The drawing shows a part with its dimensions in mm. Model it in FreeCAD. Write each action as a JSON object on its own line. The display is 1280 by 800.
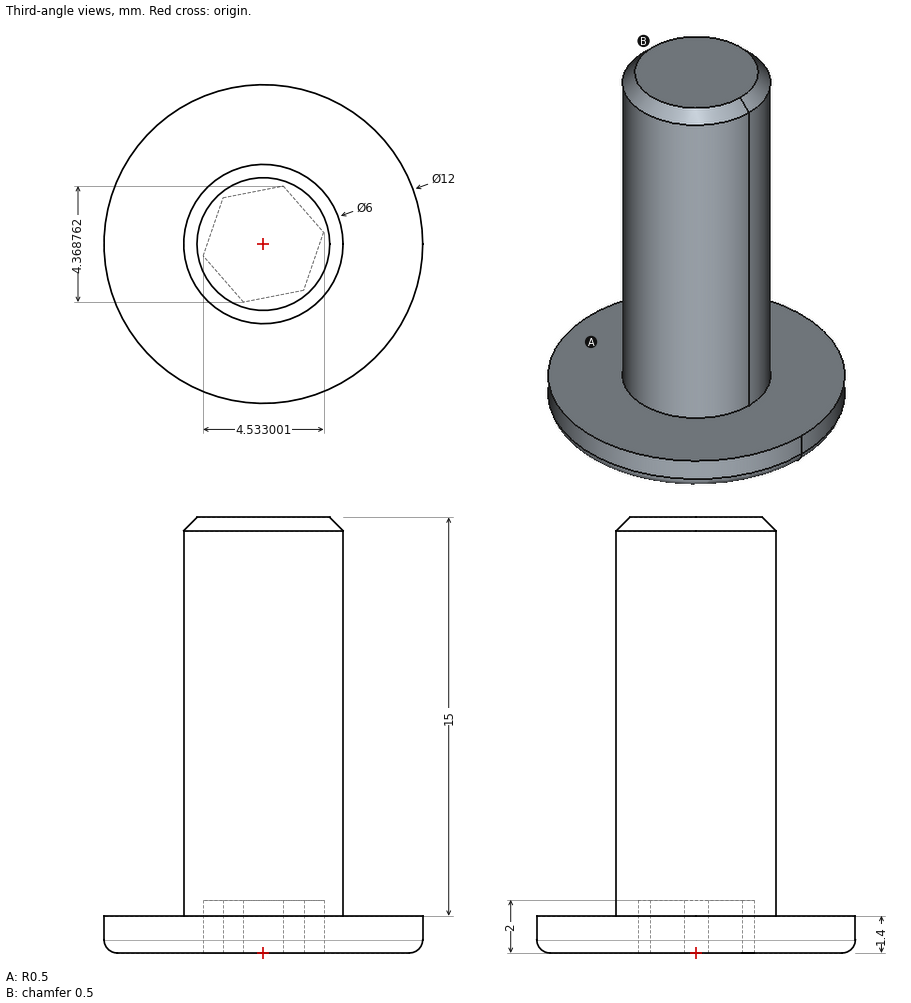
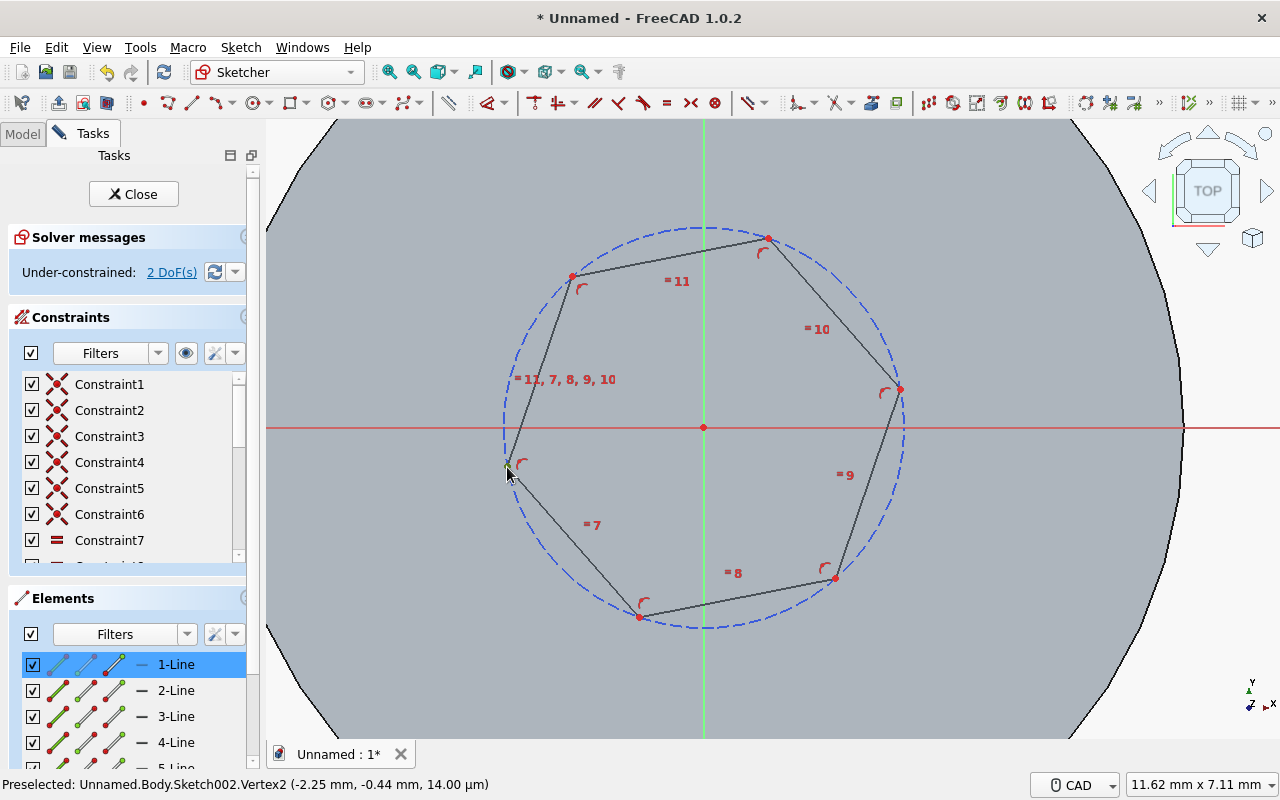
{"action": "left_click", "coordinate": [900, 389]}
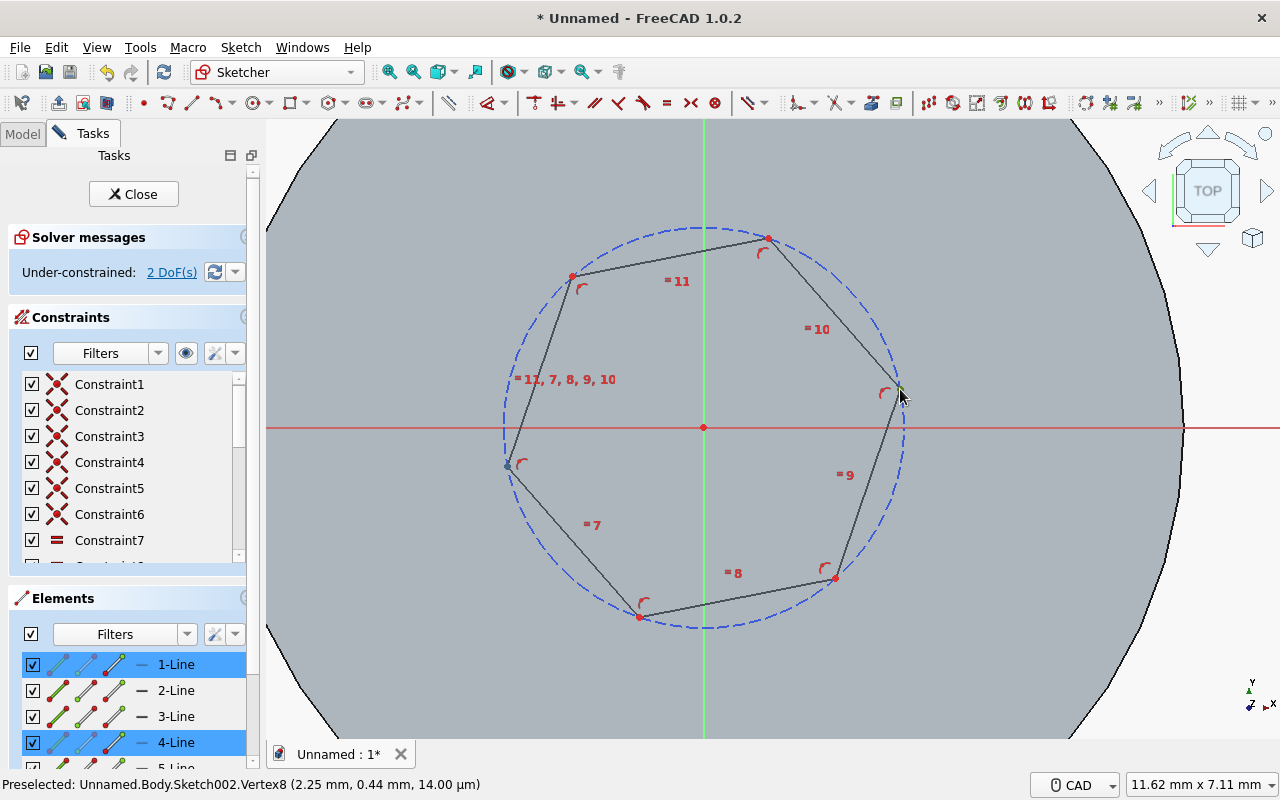
{"action": "key", "text": "l"}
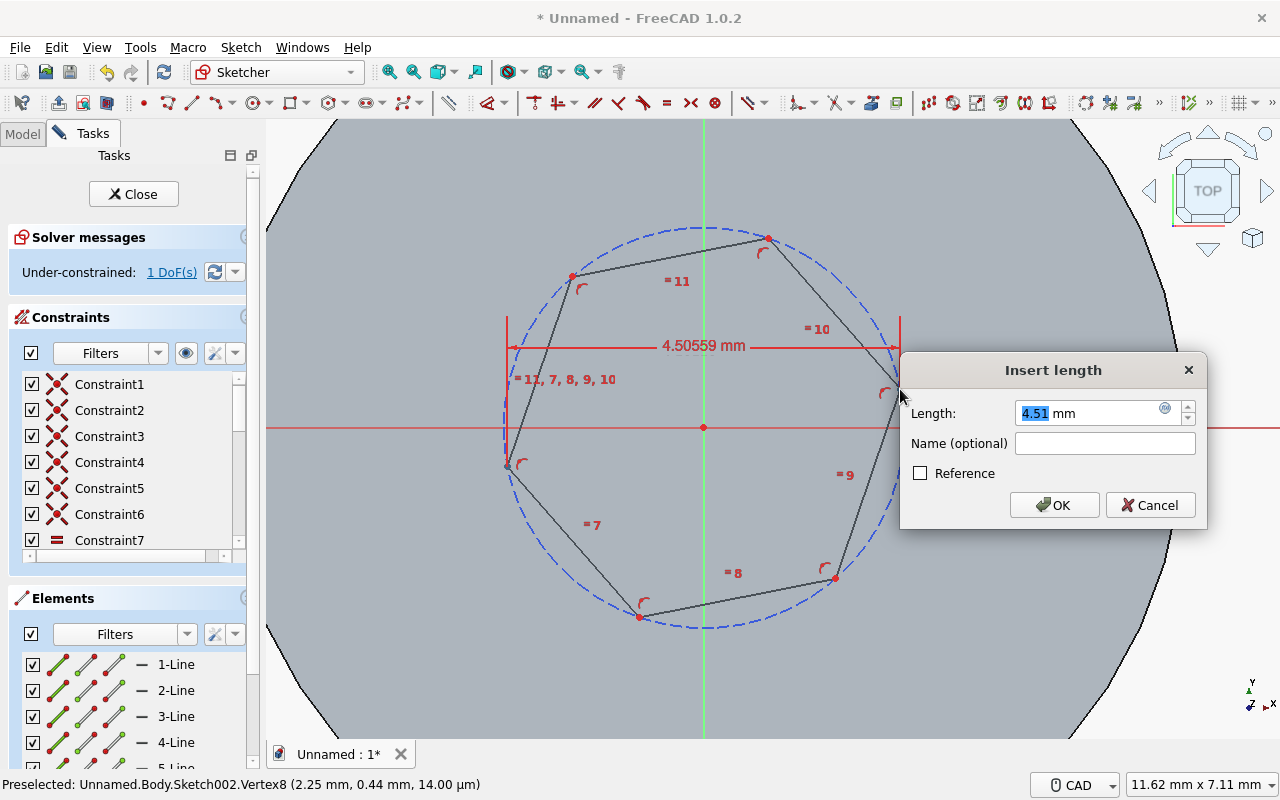
{"action": "type", "text": "4.533001"}
{"action": "key", "text": "Return"}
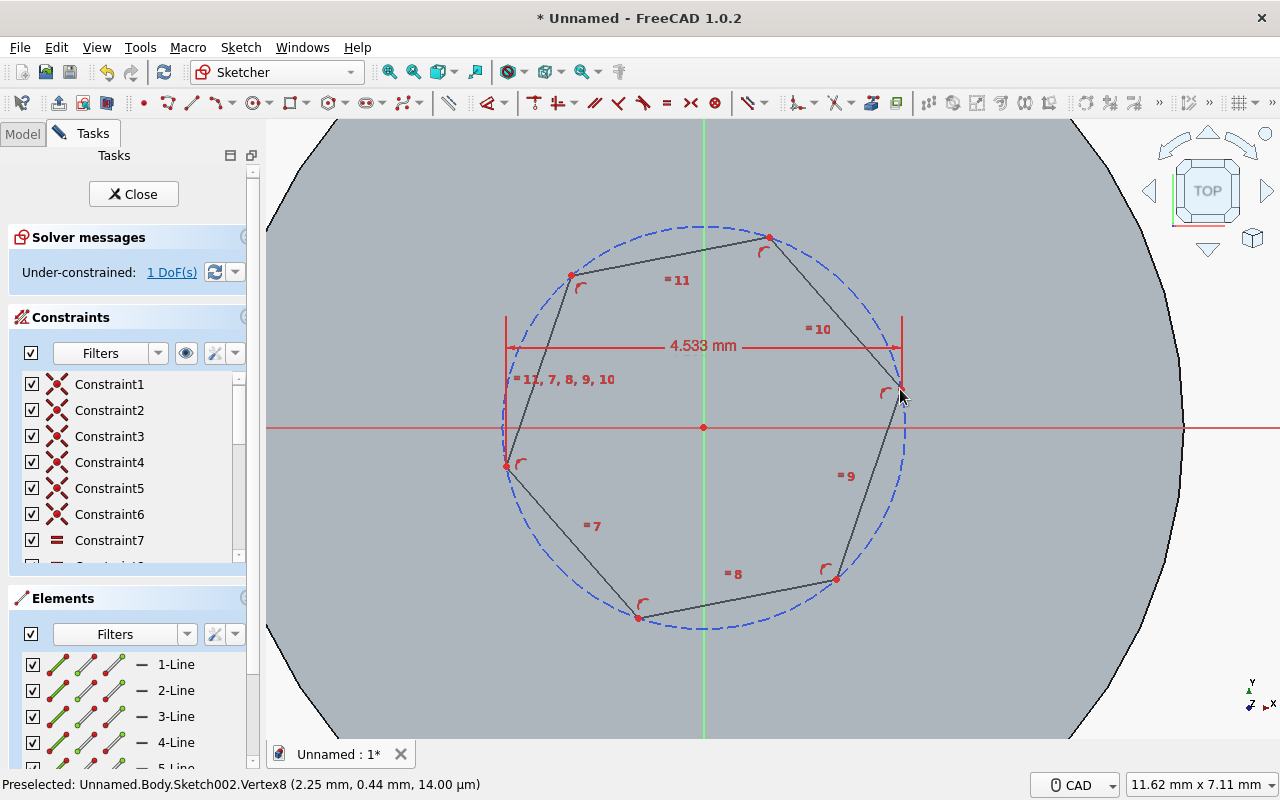
{"action": "left_click", "coordinate": [639, 619]}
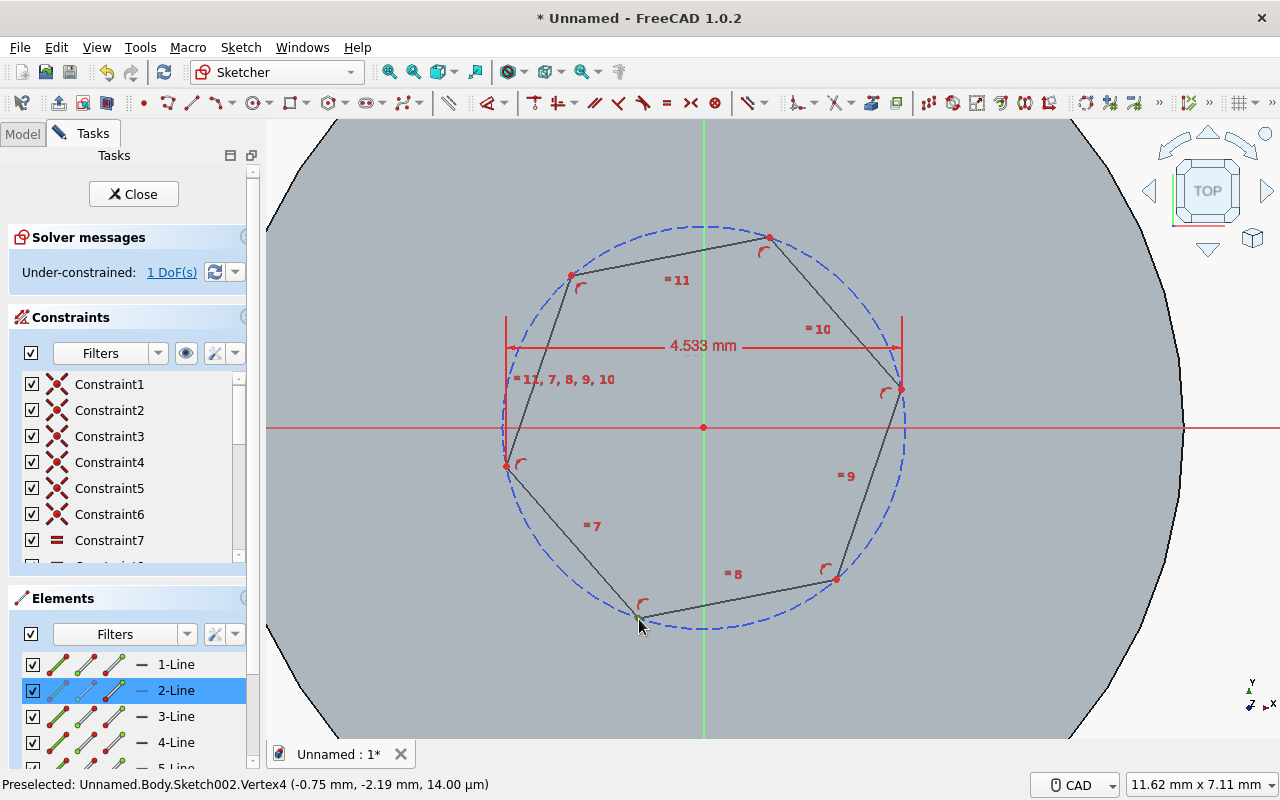
{"action": "left_click", "coordinate": [769, 237]}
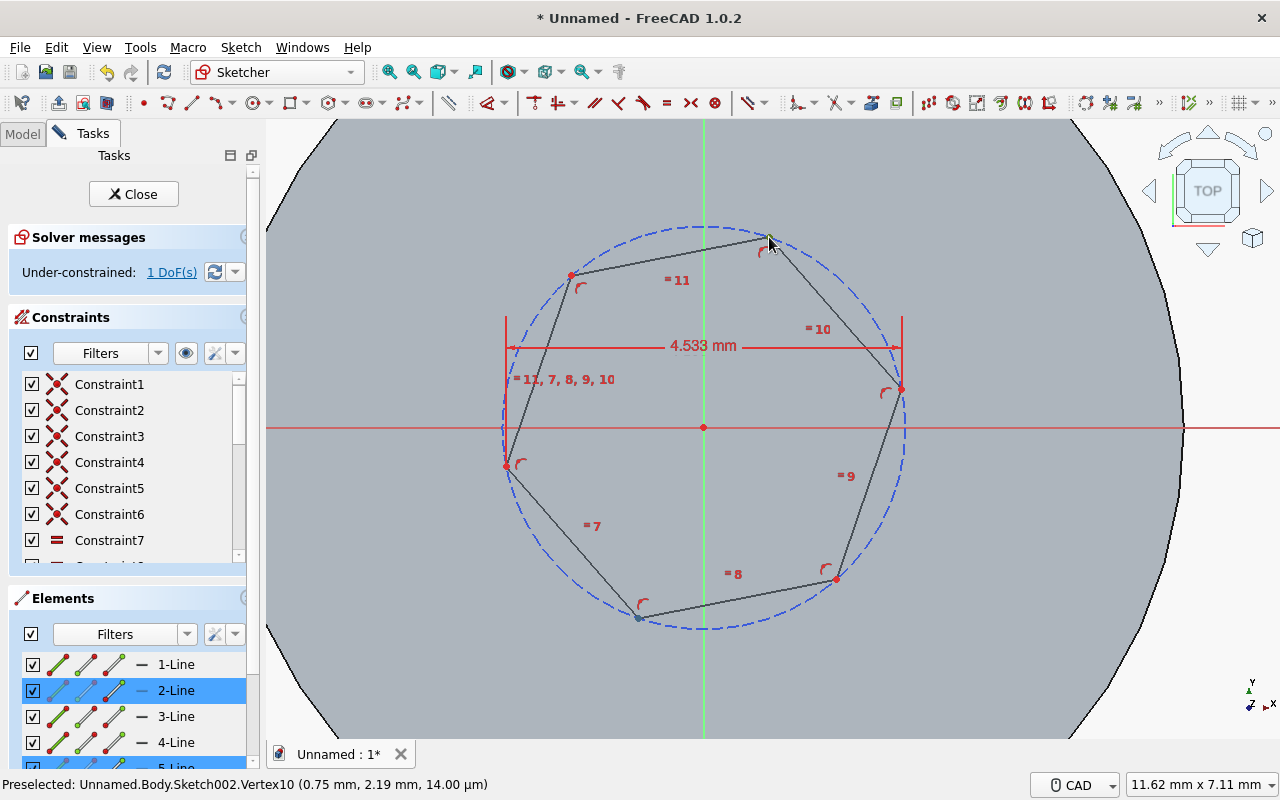
{"action": "left_click", "coordinate": [506, 104]}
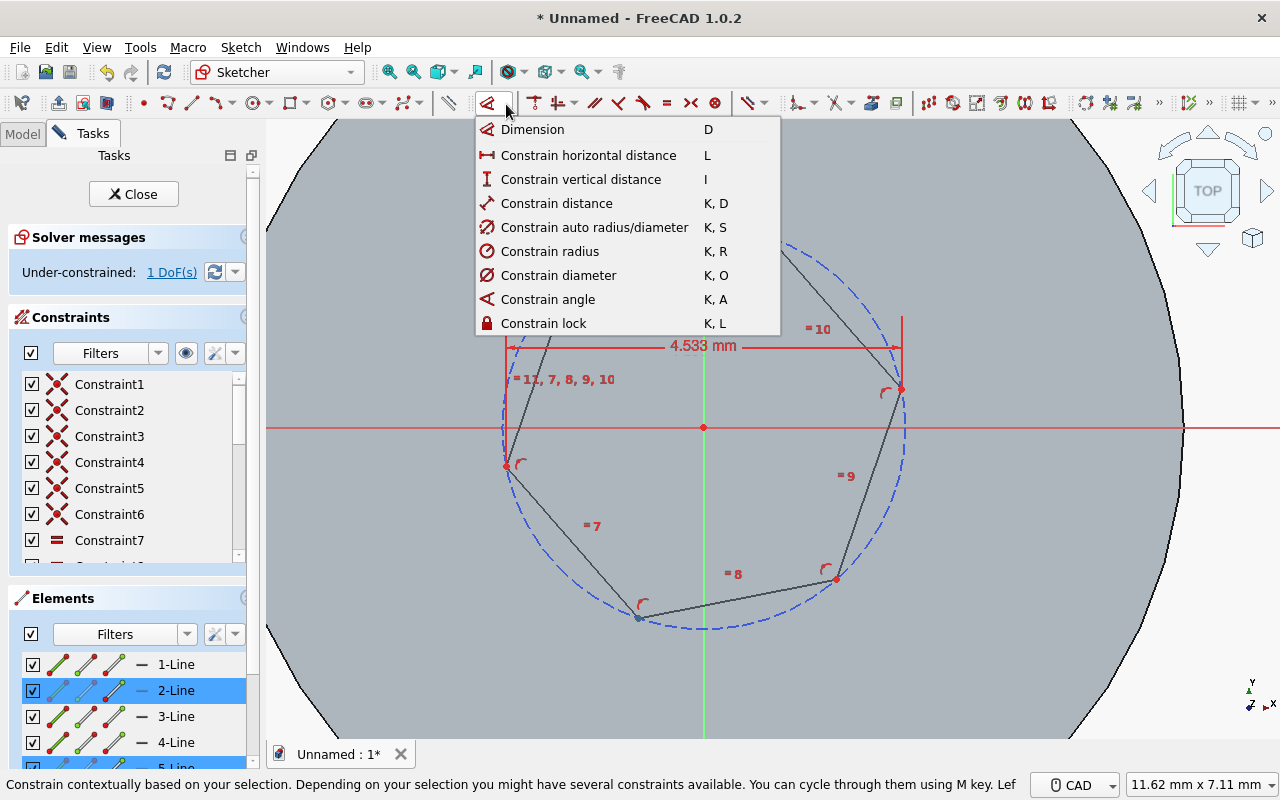
{"action": "left_click", "coordinate": [628, 179]}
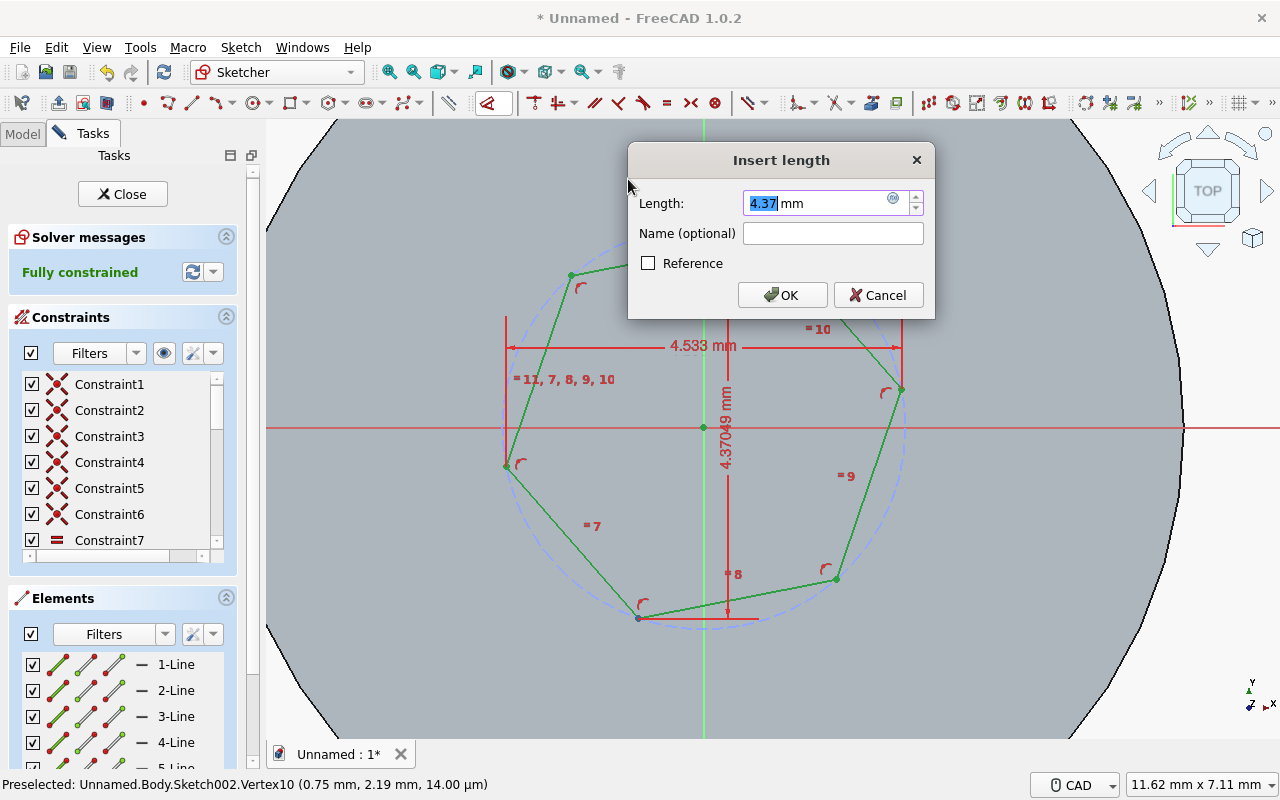
{"action": "type", "text": "4.368762"}
{"action": "key", "text": "Return"}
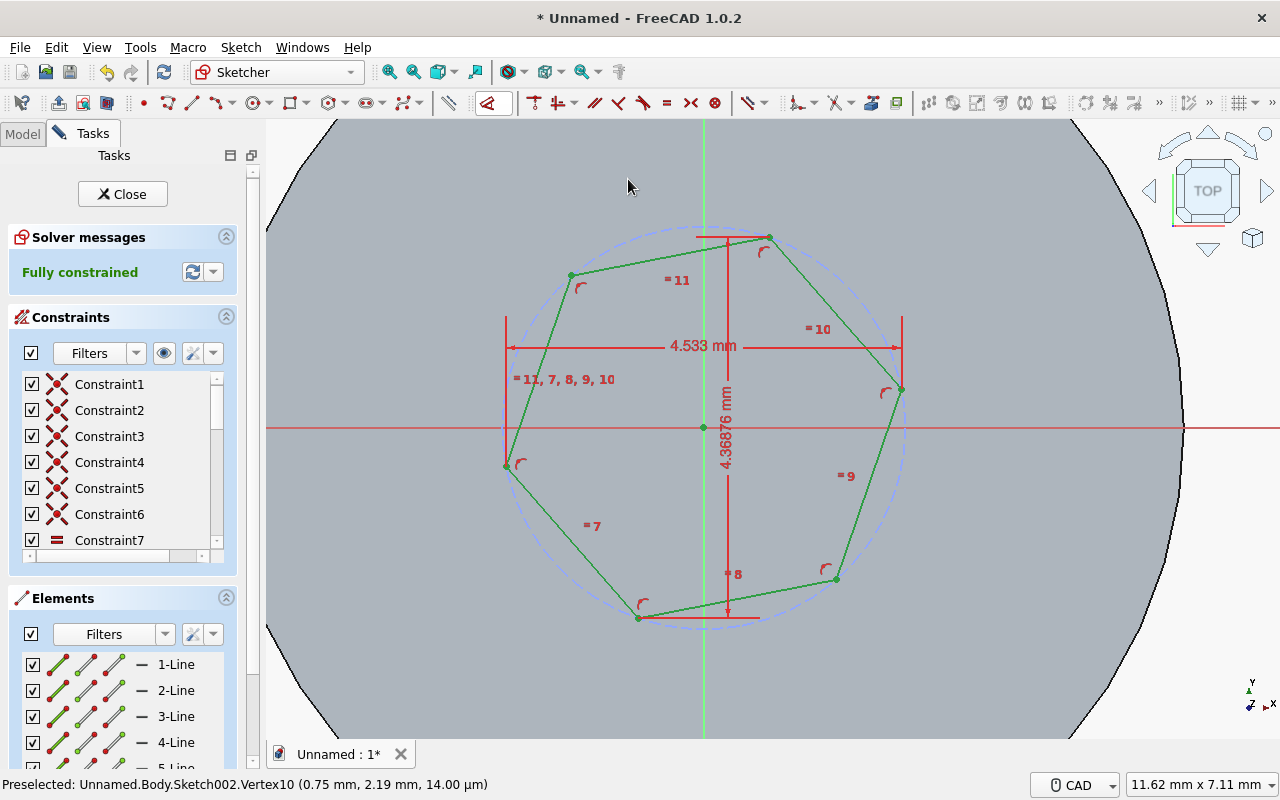
{"action": "left_click", "coordinate": [123, 194]}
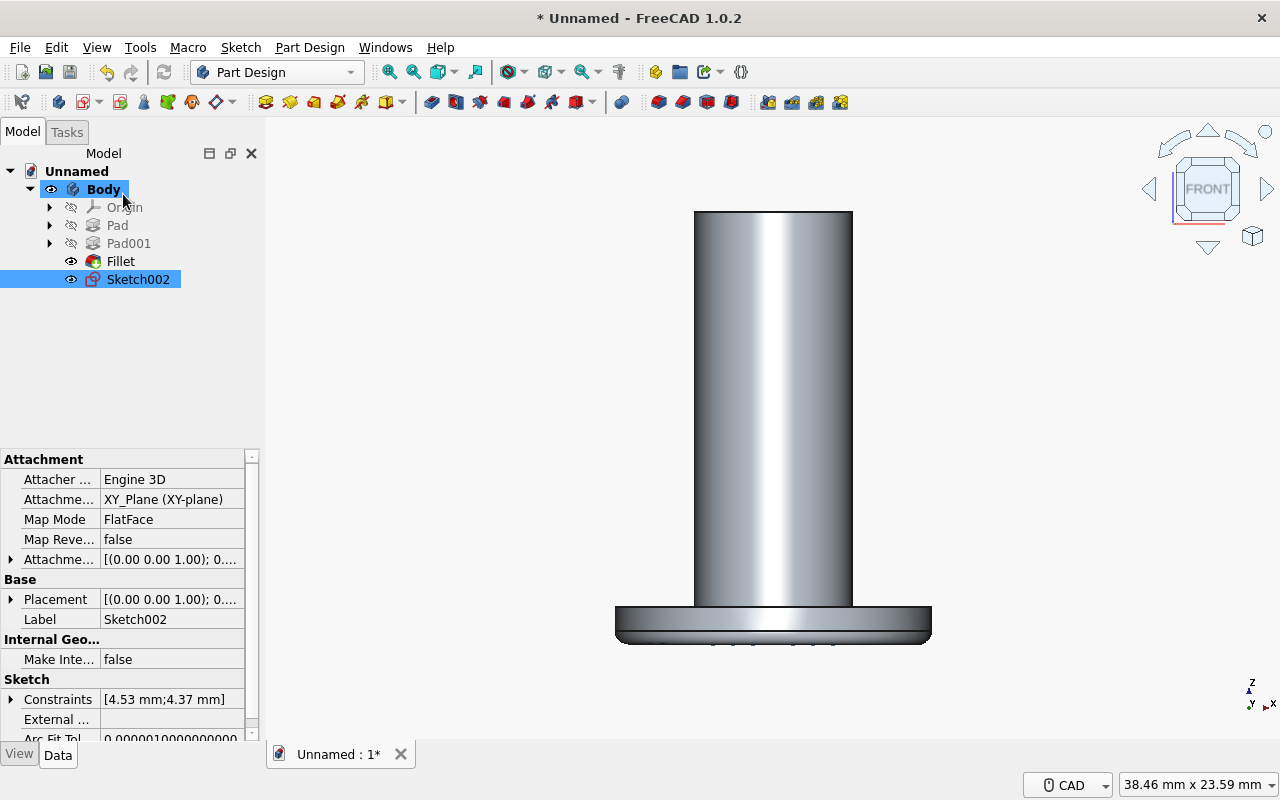
{"action": "left_click", "coordinate": [432, 102]}